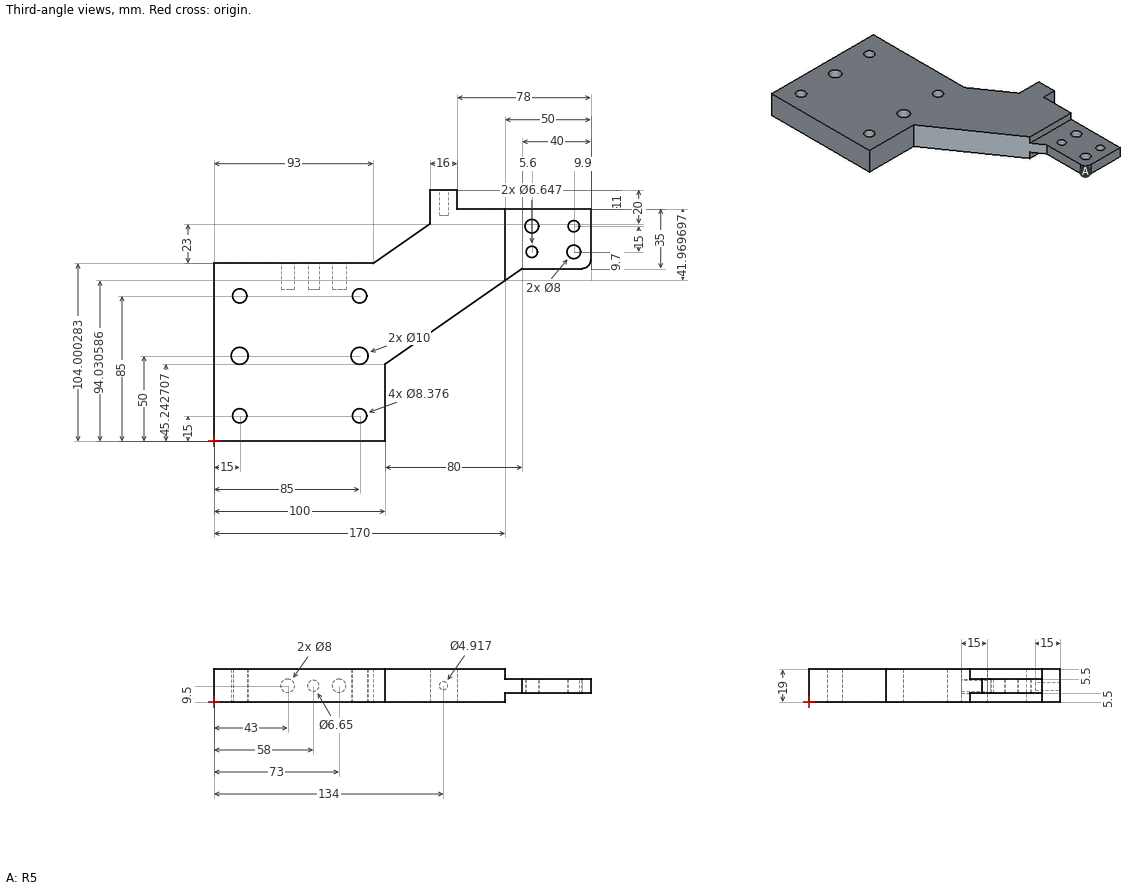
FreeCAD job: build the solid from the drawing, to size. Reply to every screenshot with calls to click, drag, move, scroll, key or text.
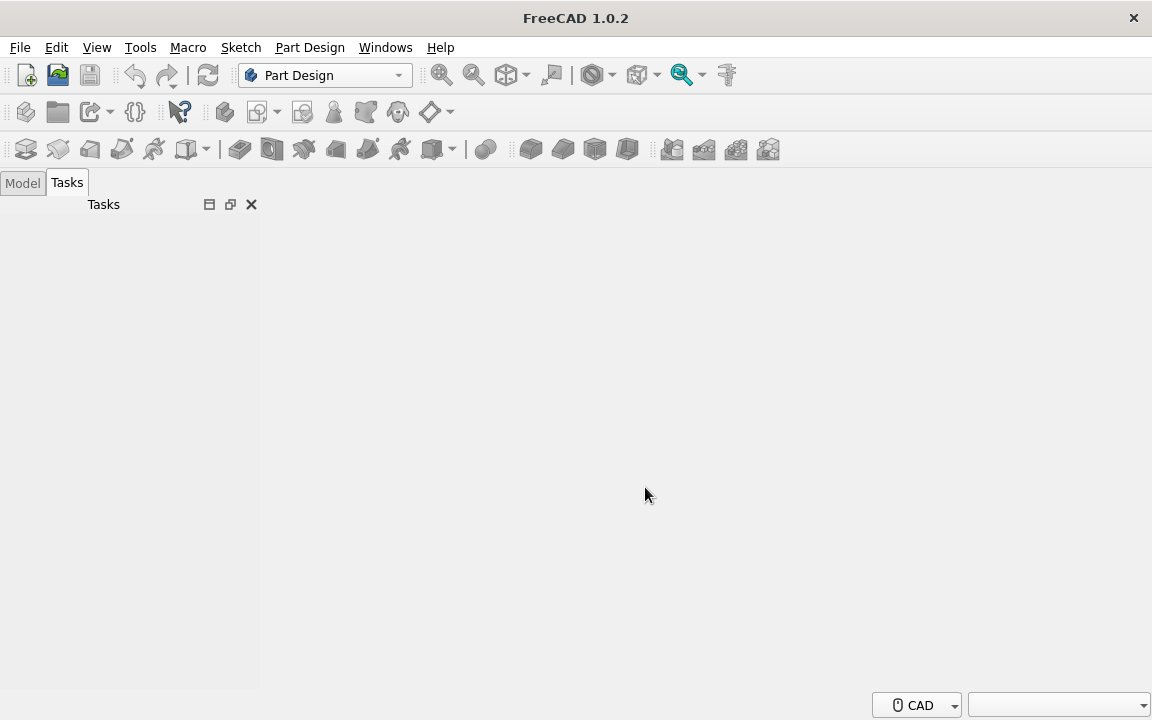
click(26, 76)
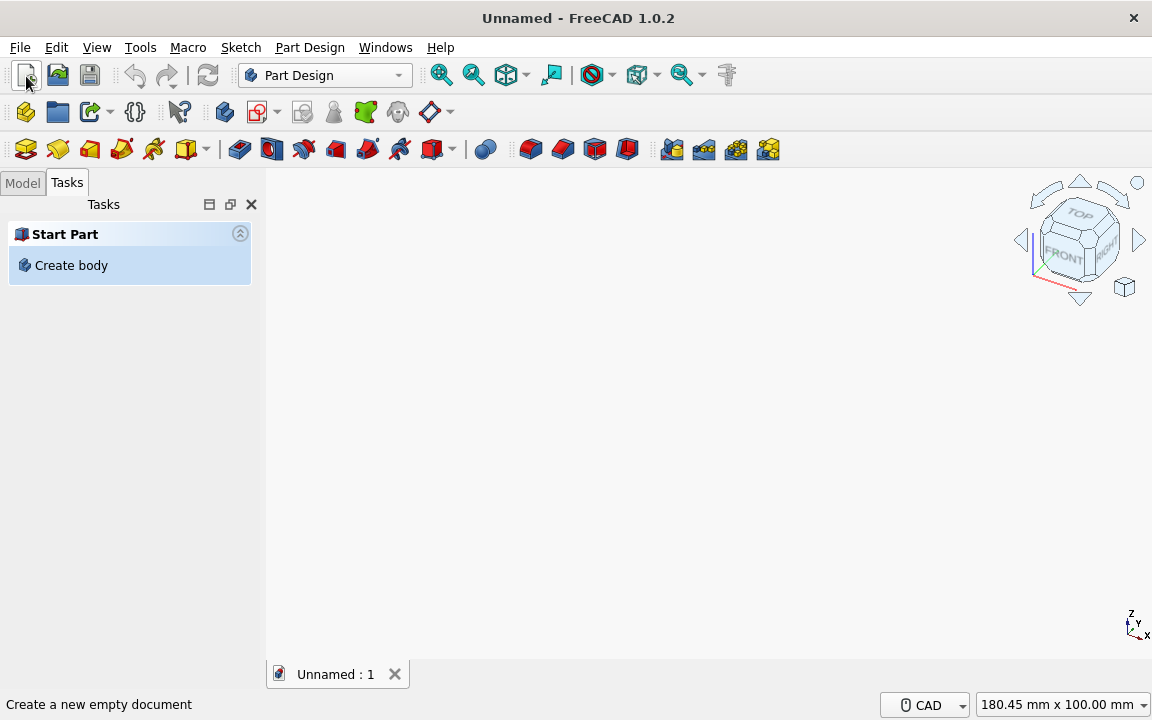
click(258, 112)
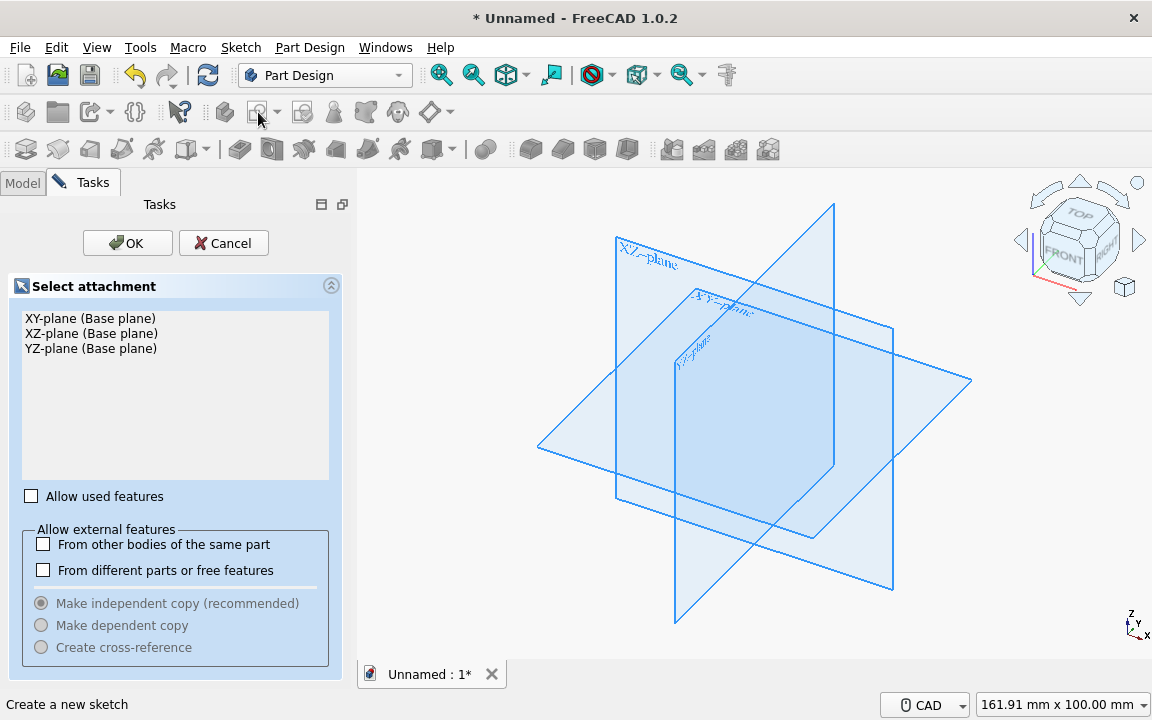
click(82, 318)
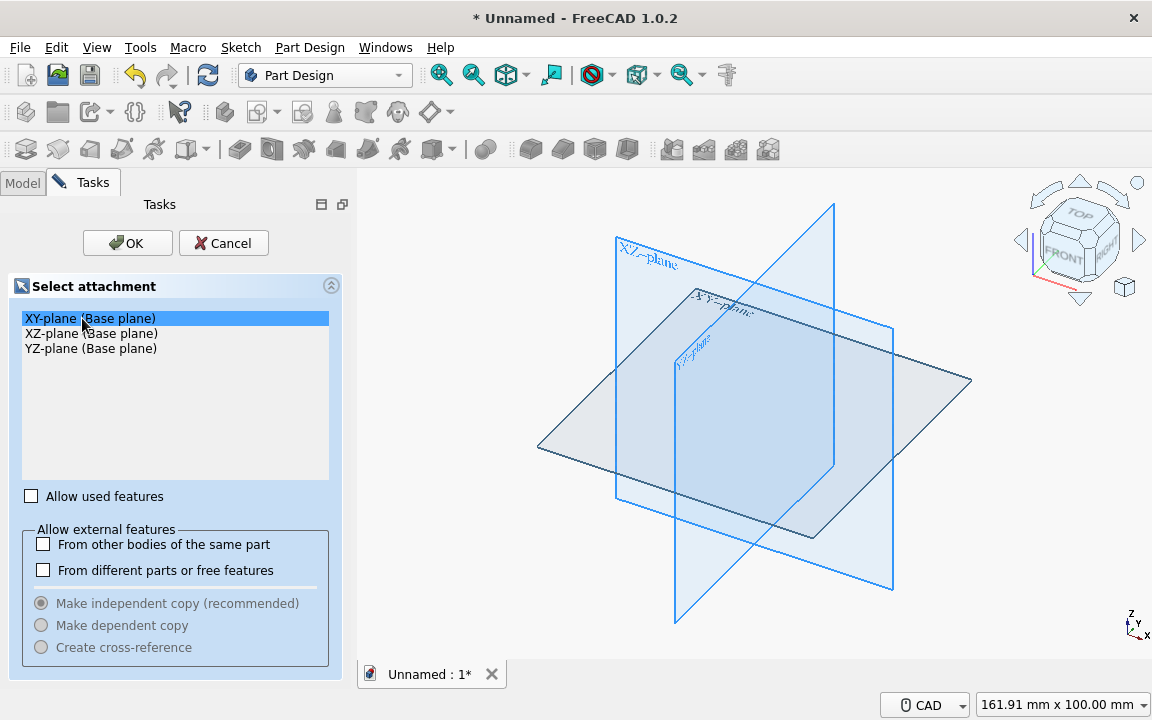
click(128, 243)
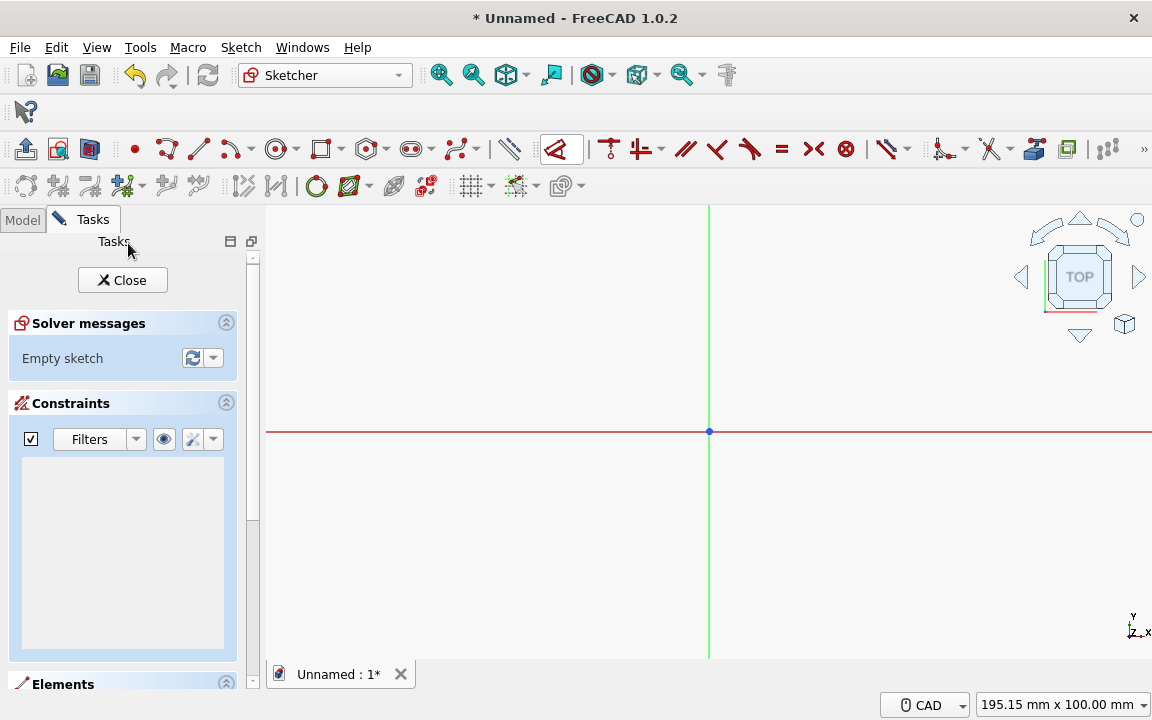
scroll(310, 626, down, 5)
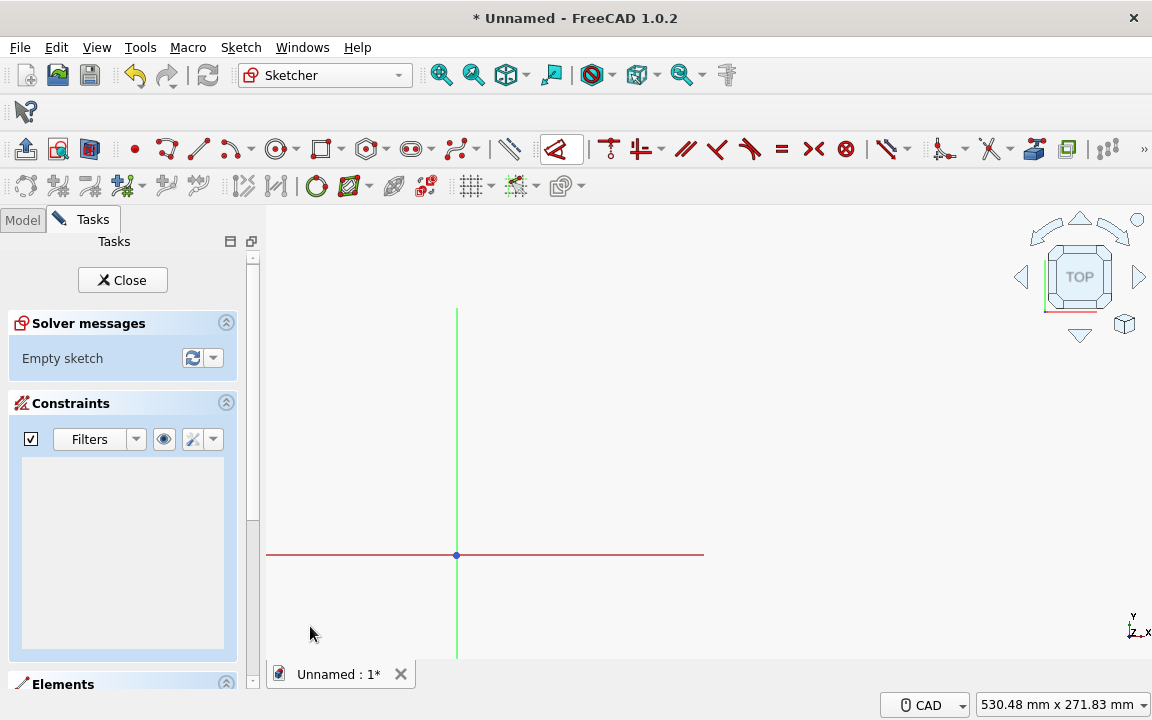
click(168, 150)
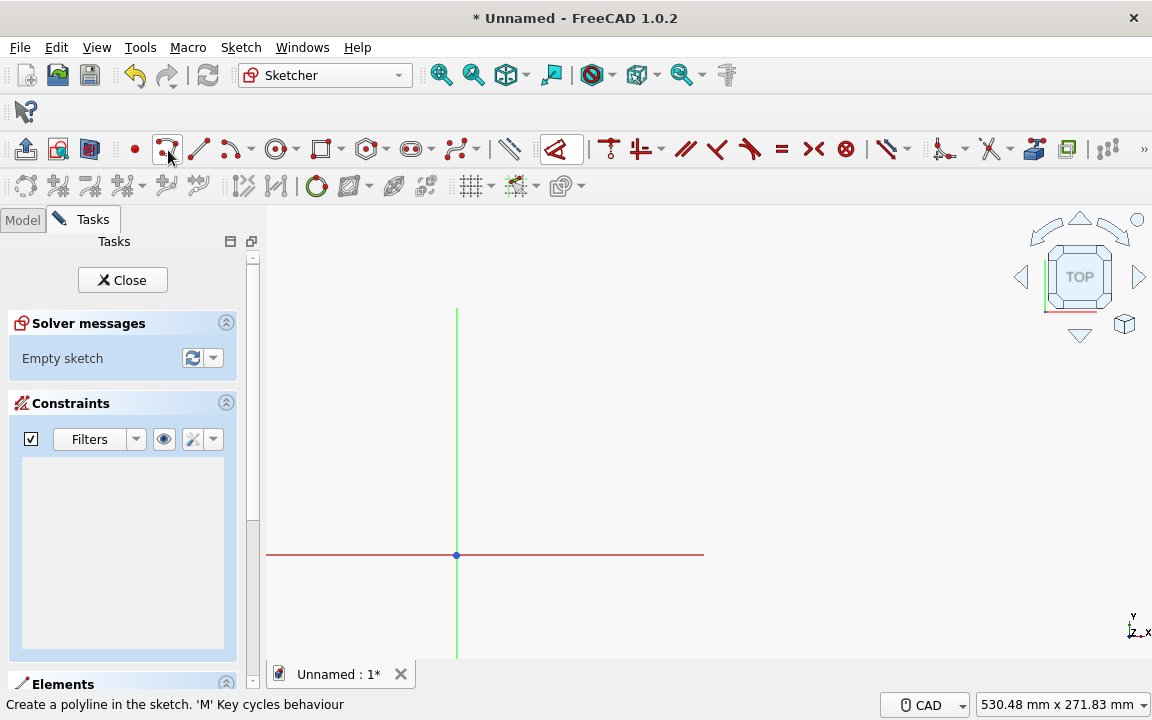
click(457, 555)
click(624, 546)
click(624, 480)
click(757, 387)
click(824, 387)
click(824, 328)
click(694, 328)
click(694, 310)
click(667, 310)
click(667, 343)
click(612, 382)
click(466, 382)
click(457, 555)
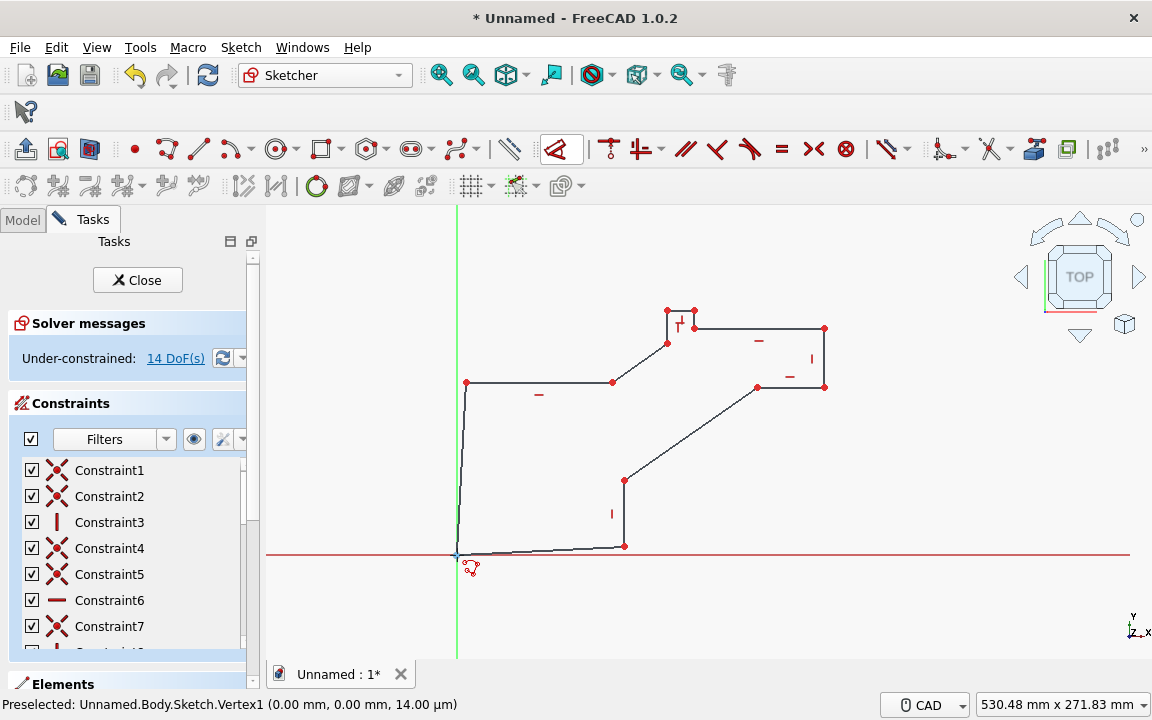
click(276, 150)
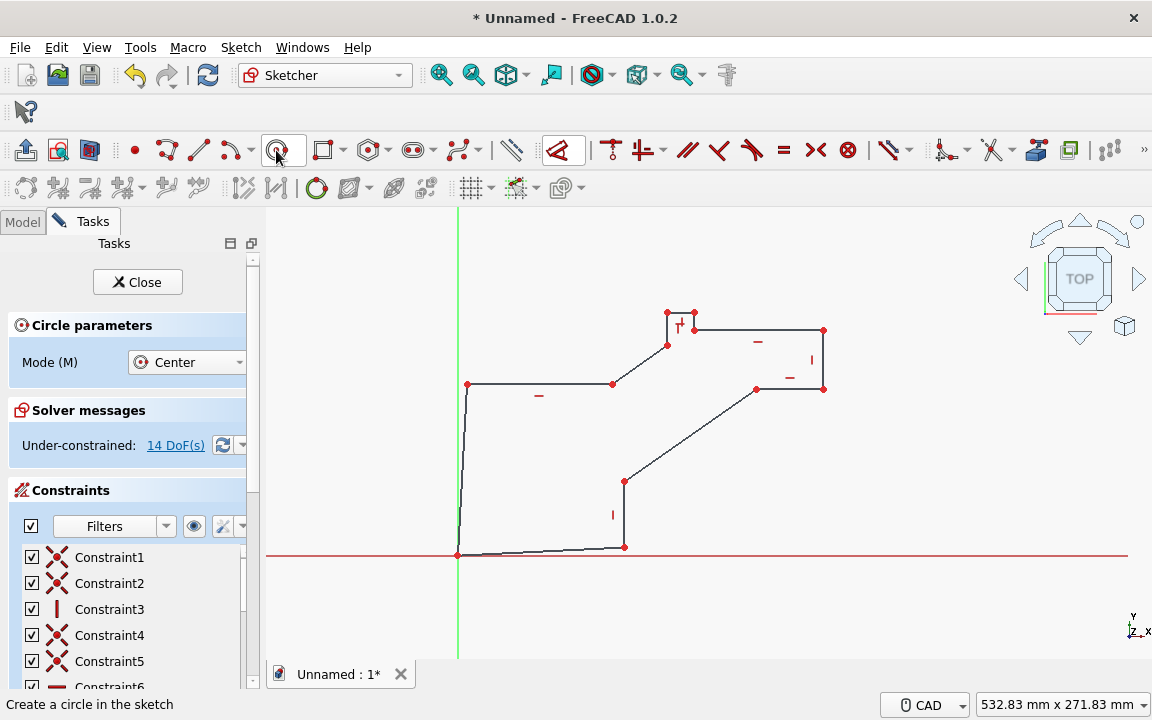
scroll(599, 531, up, 6)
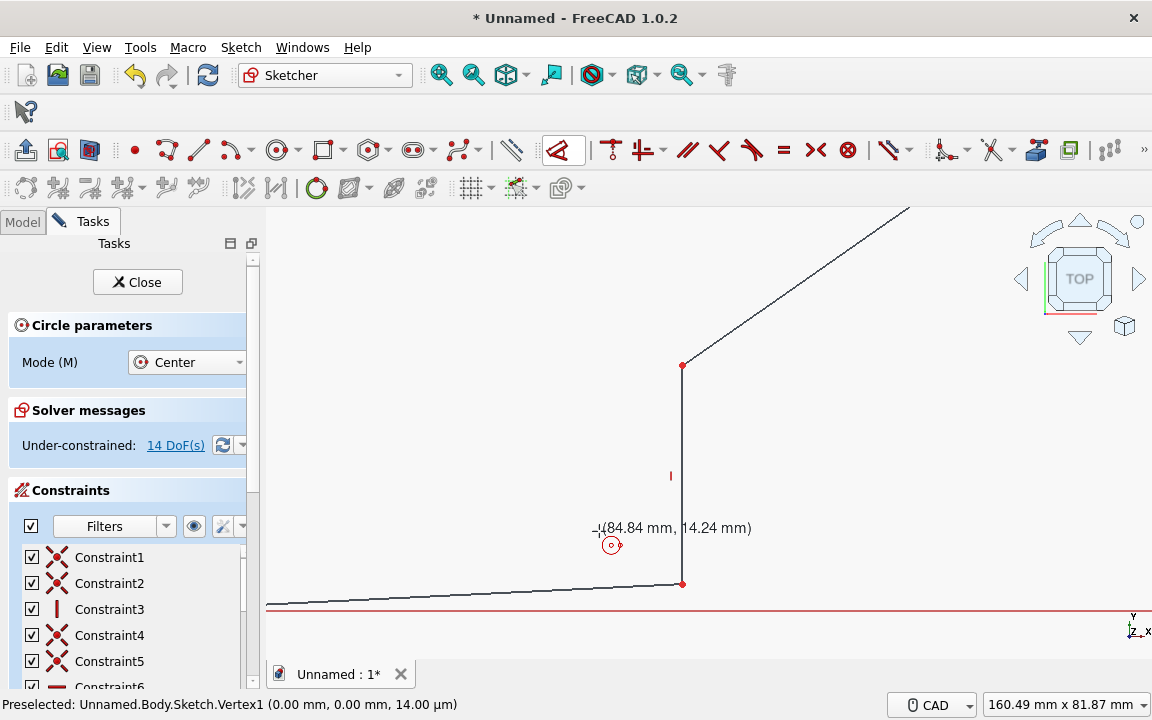
click(599, 528)
click(615, 512)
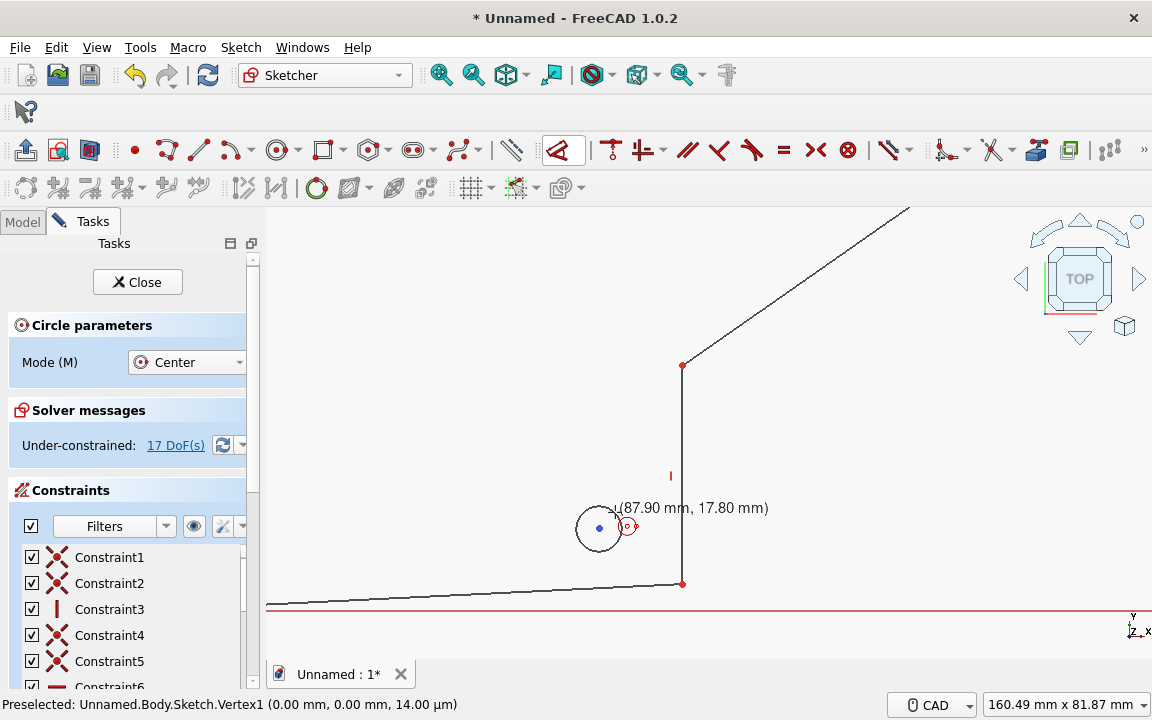
scroll(584, 565, down, 5)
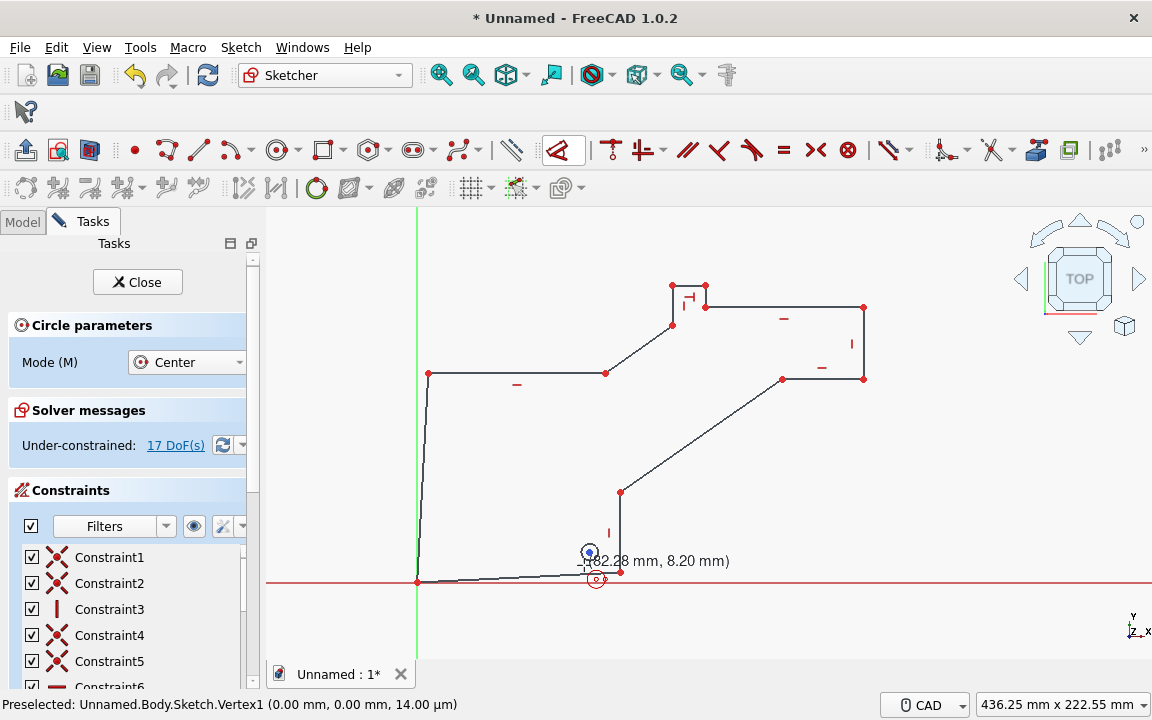
scroll(448, 552, up, 5)